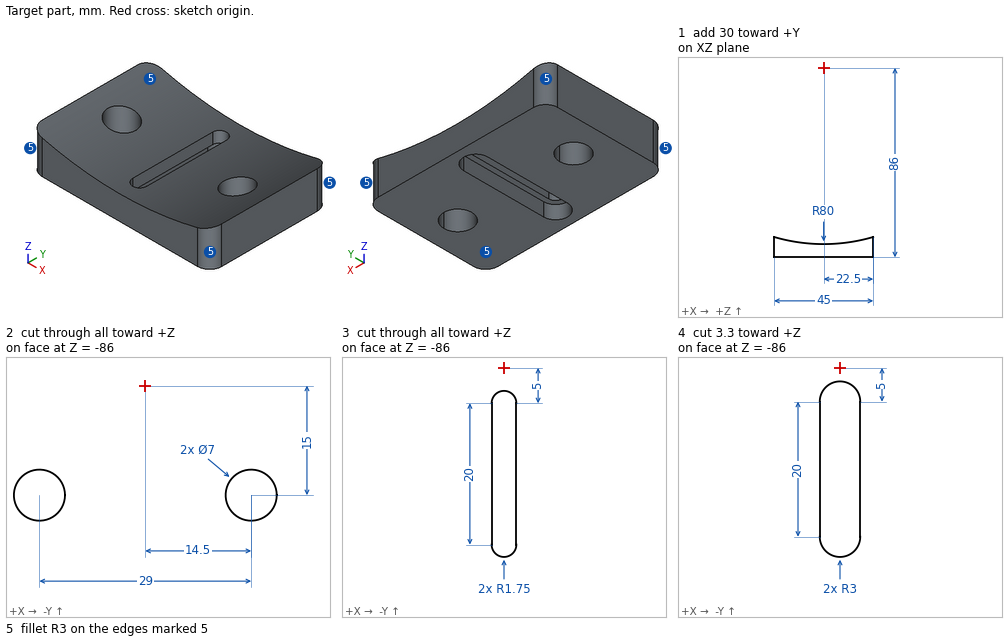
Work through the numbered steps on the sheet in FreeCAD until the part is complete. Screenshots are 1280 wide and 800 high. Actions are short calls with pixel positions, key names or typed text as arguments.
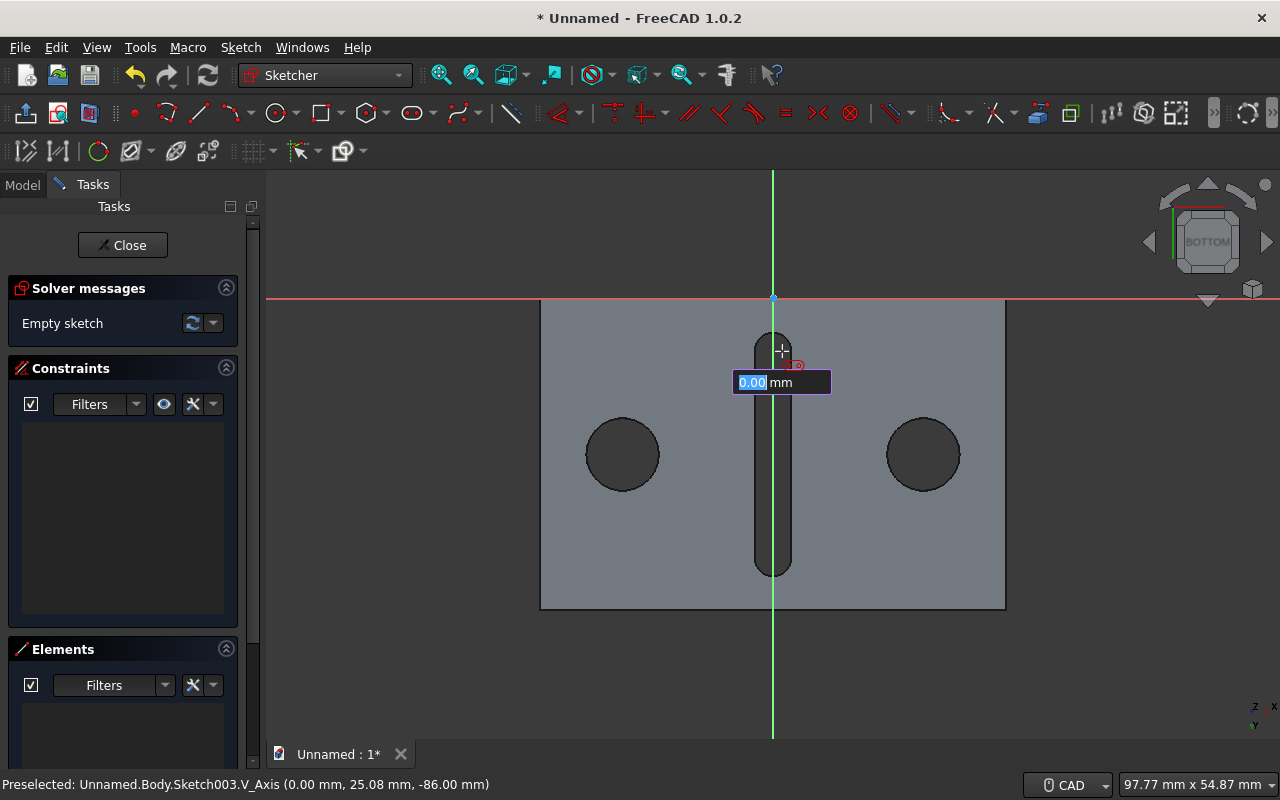
click(742, 454)
key(Escape)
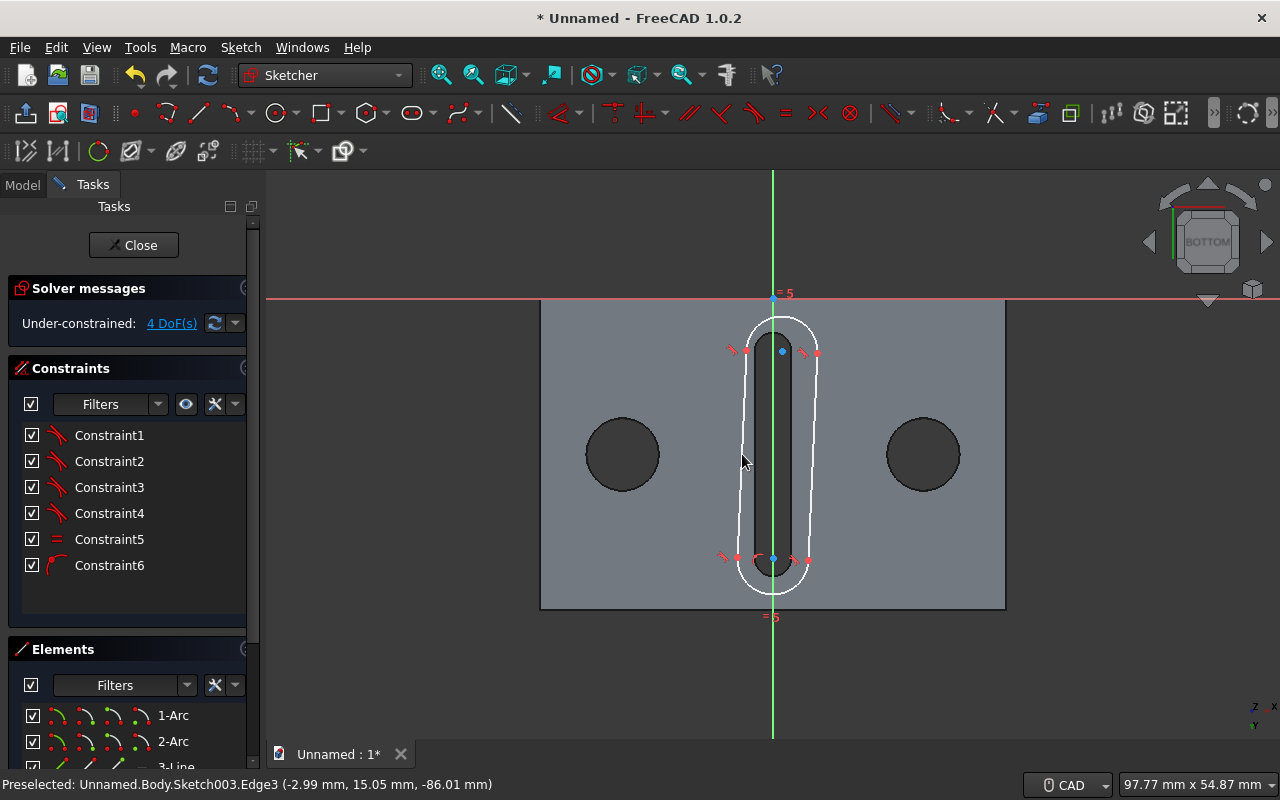
click(740, 495)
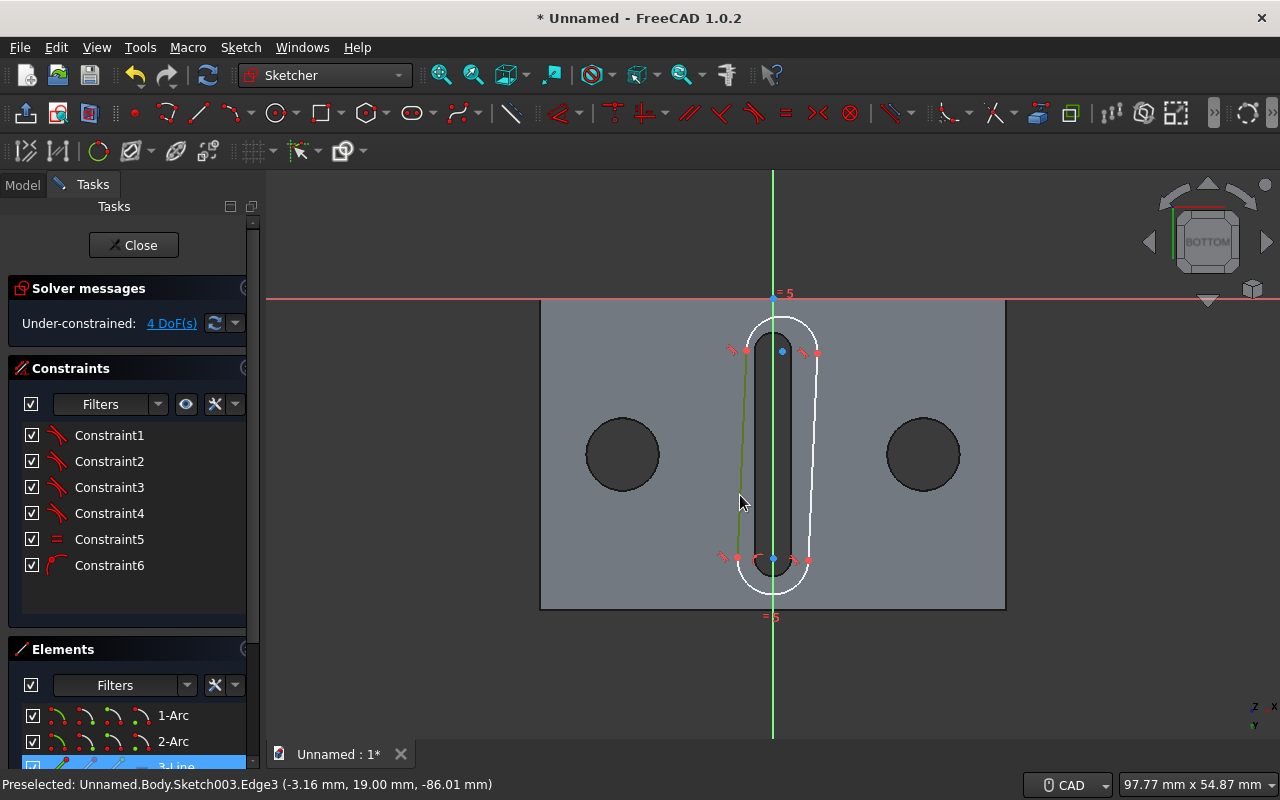
click(668, 114)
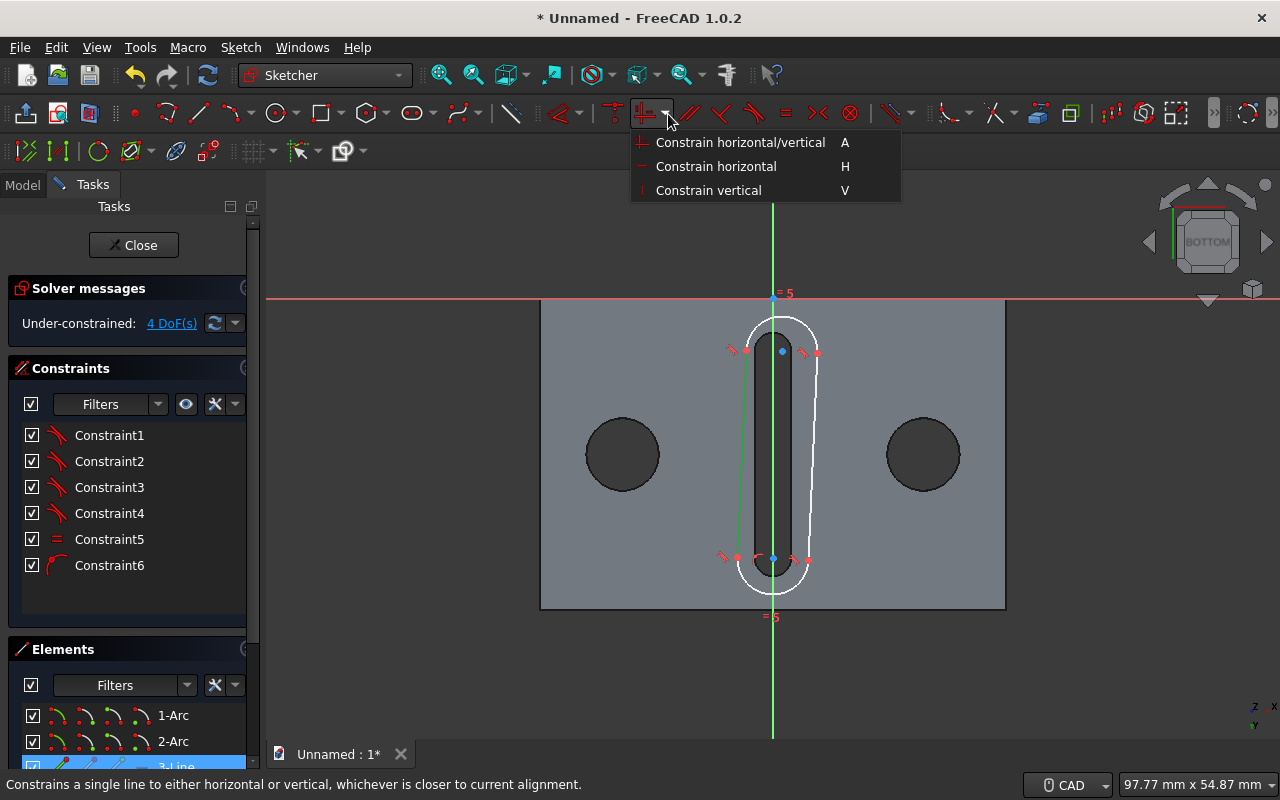
click(766, 190)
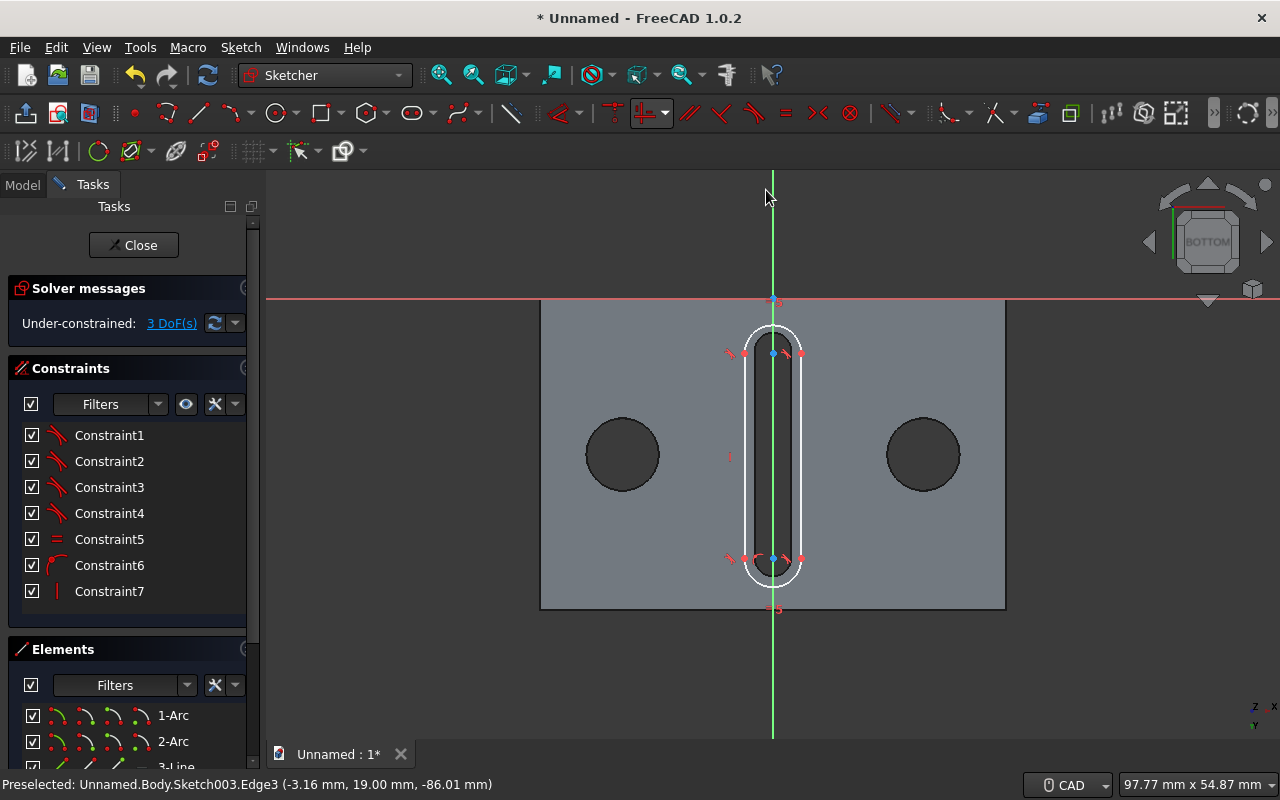
key(d)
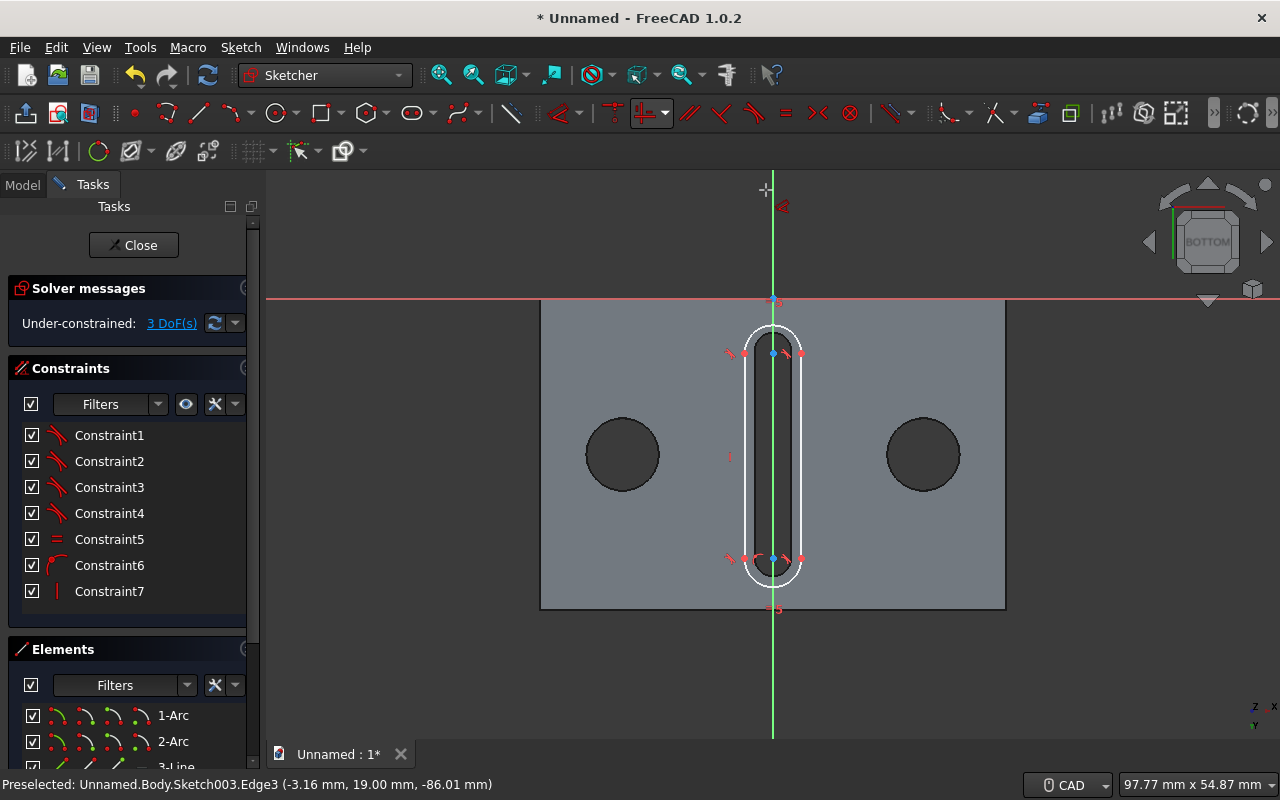
scroll(756, 582, up, 2)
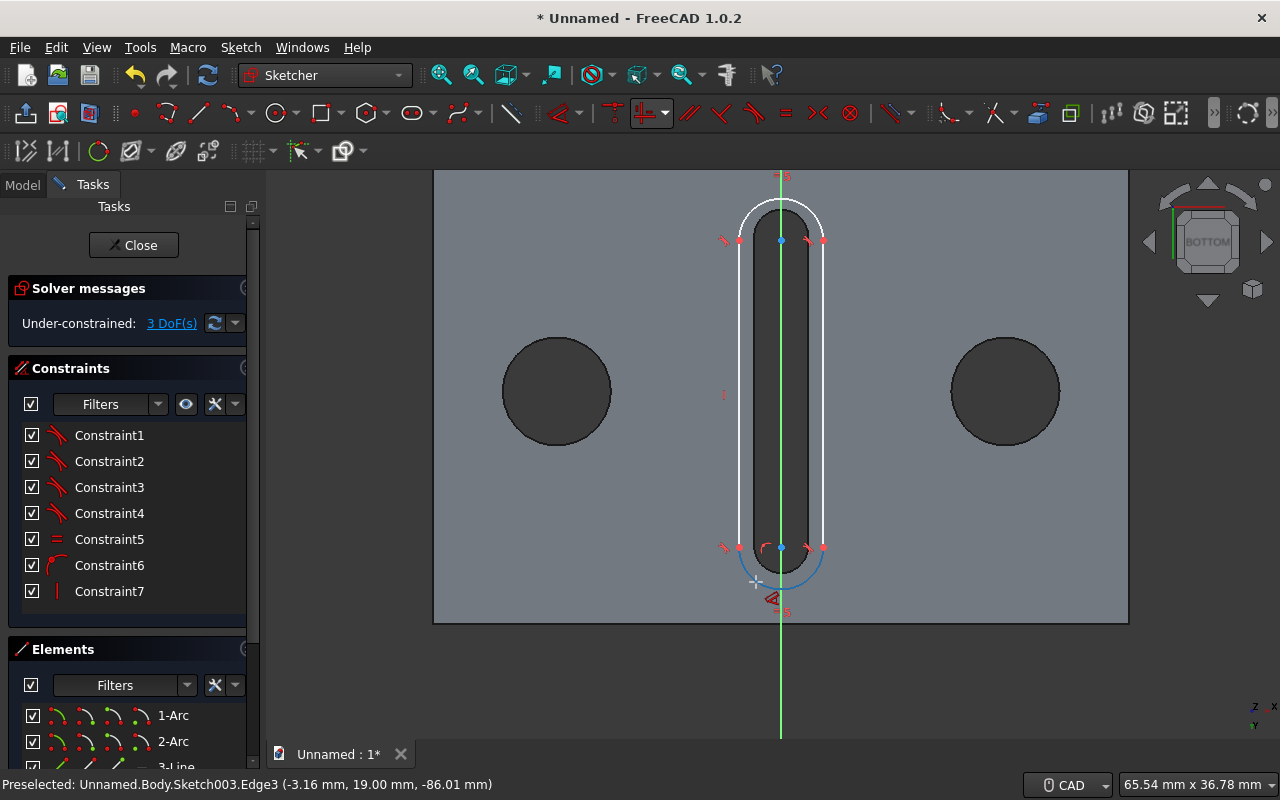
click(756, 581)
click(737, 607)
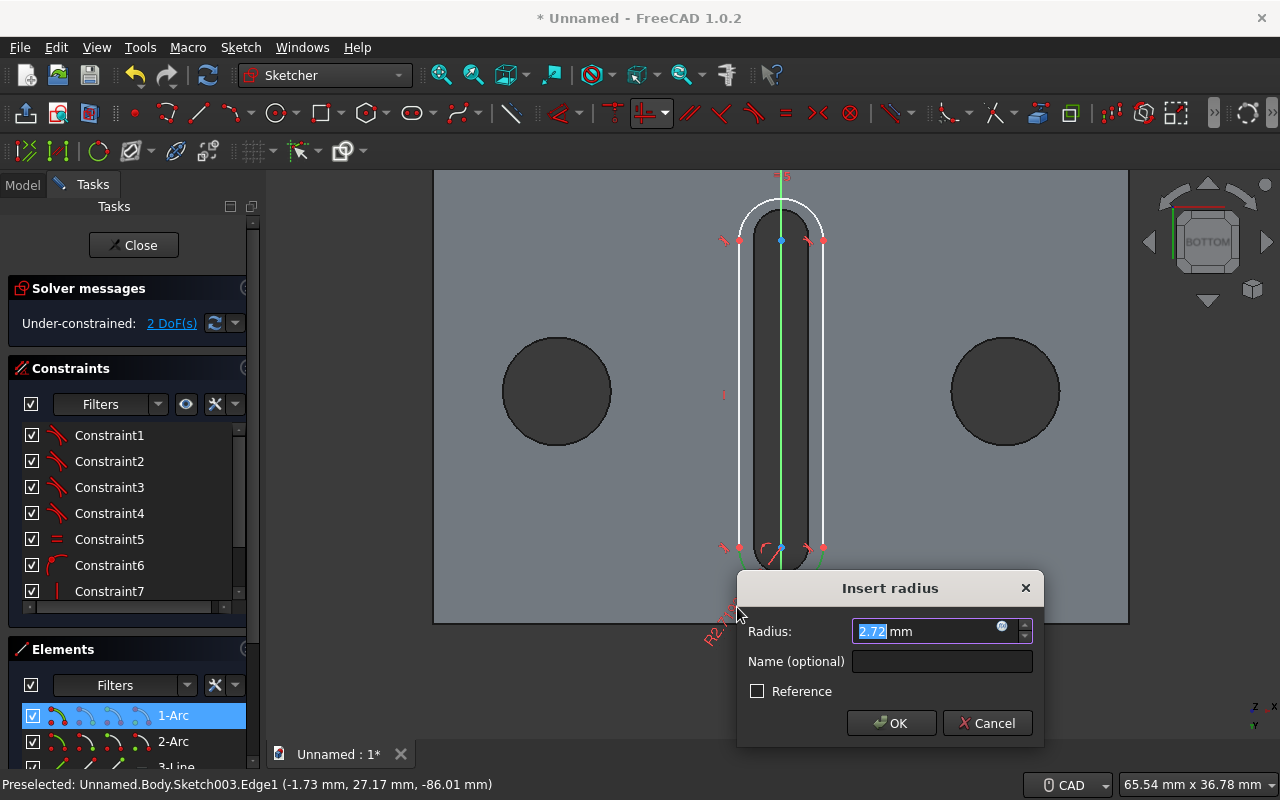
text(3)
key(Return)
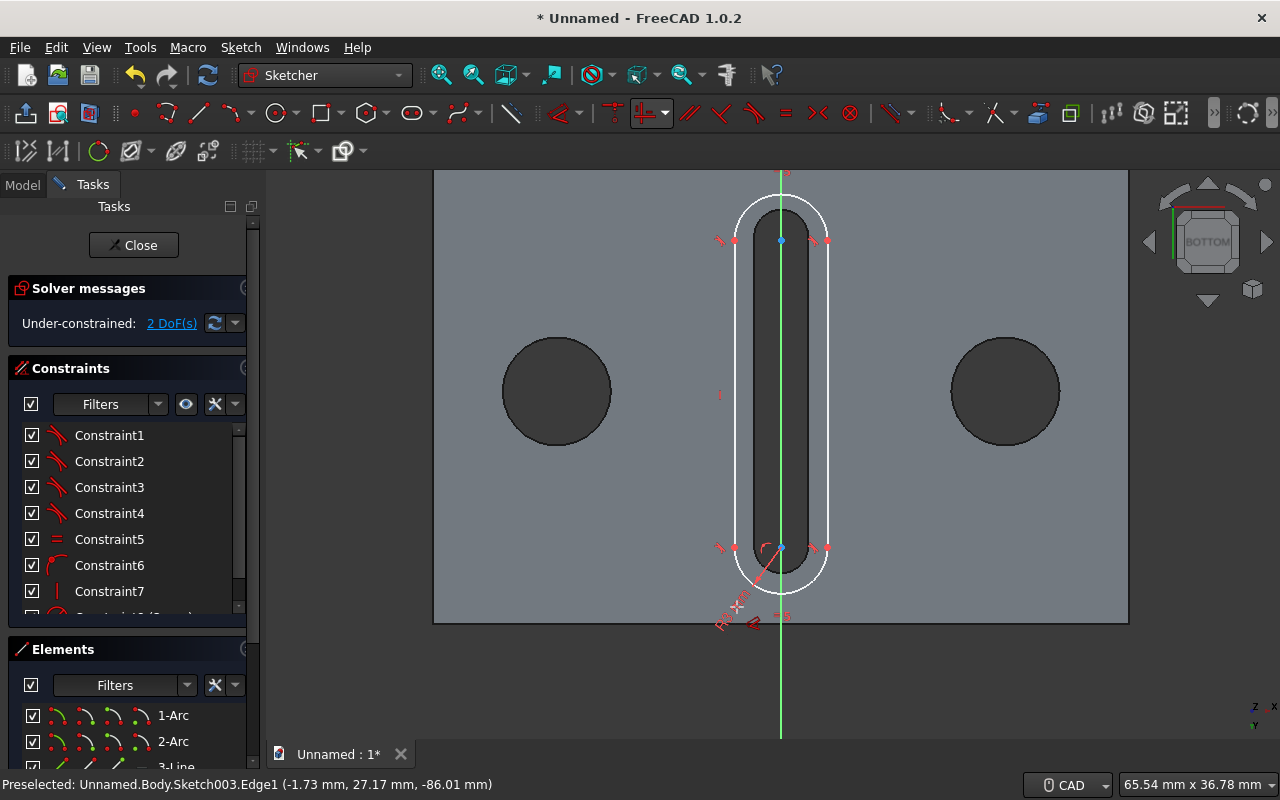
click(735, 455)
click(701, 394)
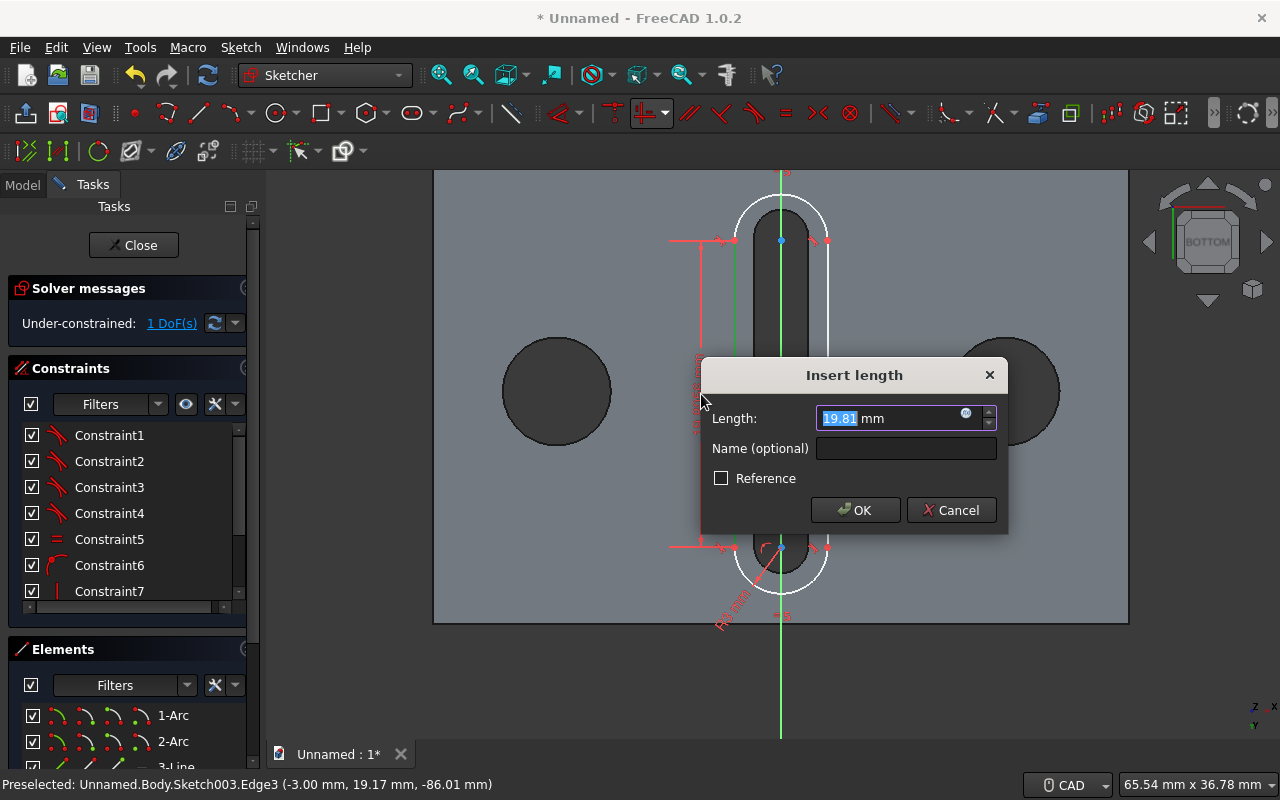
text(20)
key(Return)